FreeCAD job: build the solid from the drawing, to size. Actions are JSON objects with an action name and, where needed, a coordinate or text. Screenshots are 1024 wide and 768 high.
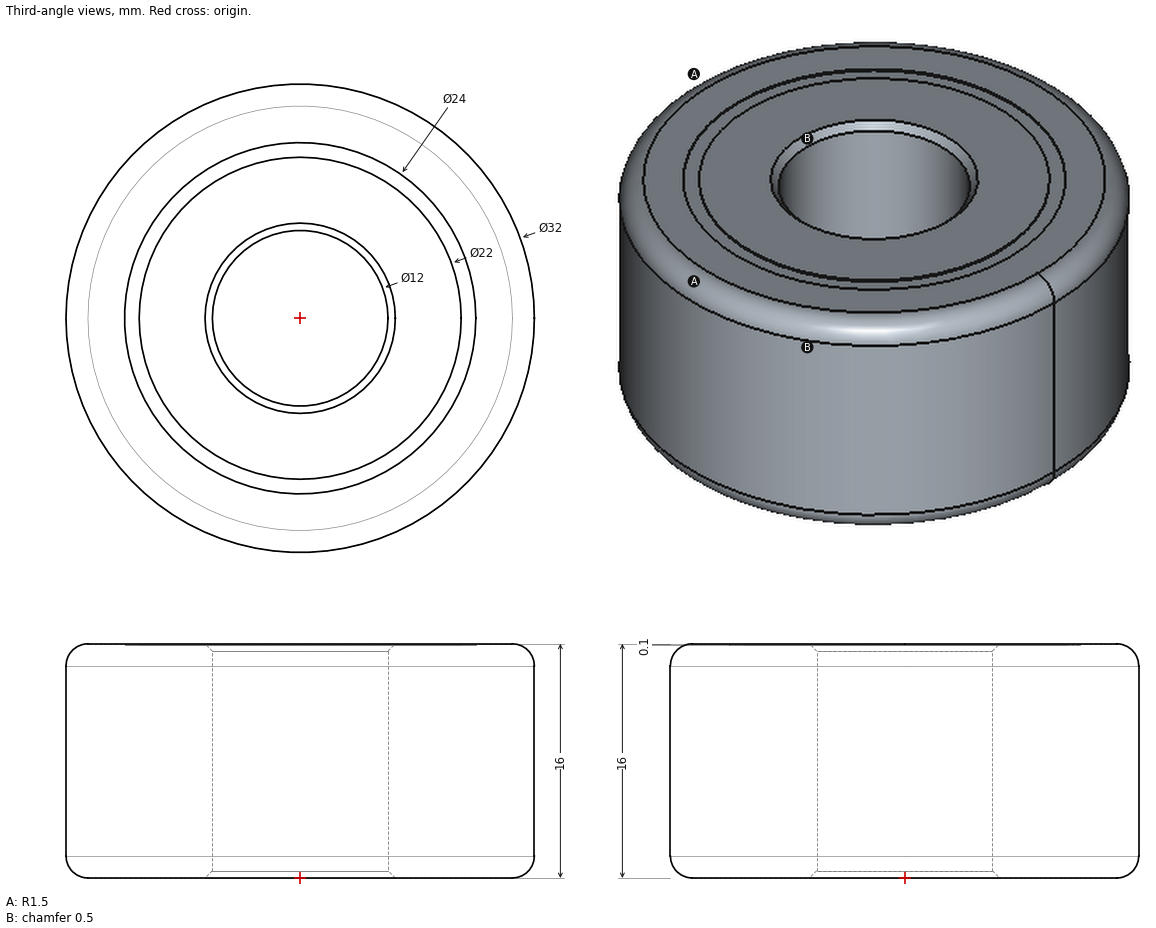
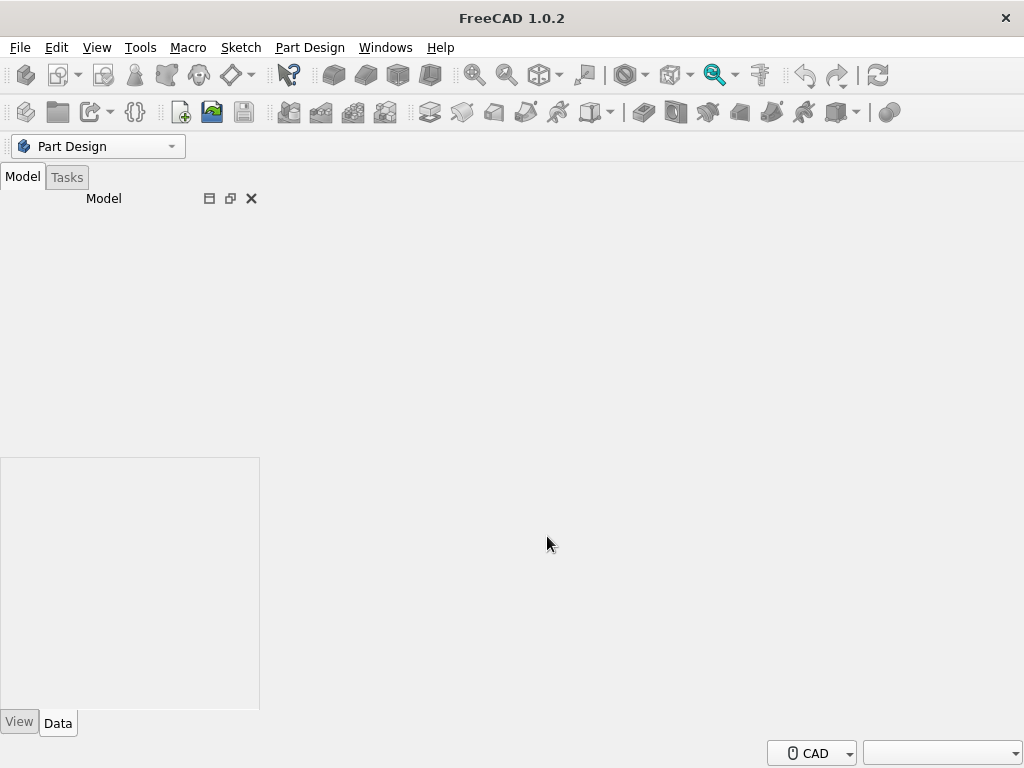
{"action": "key", "text": "ctrl+n"}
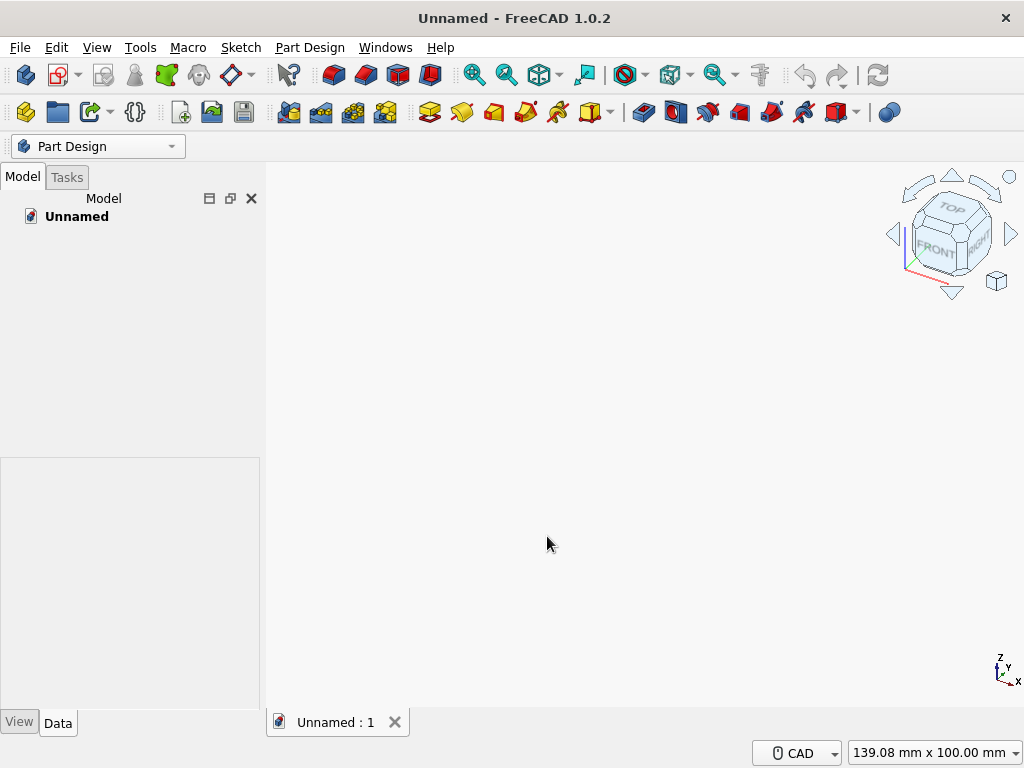
{"action": "left_click", "coordinate": [58, 76]}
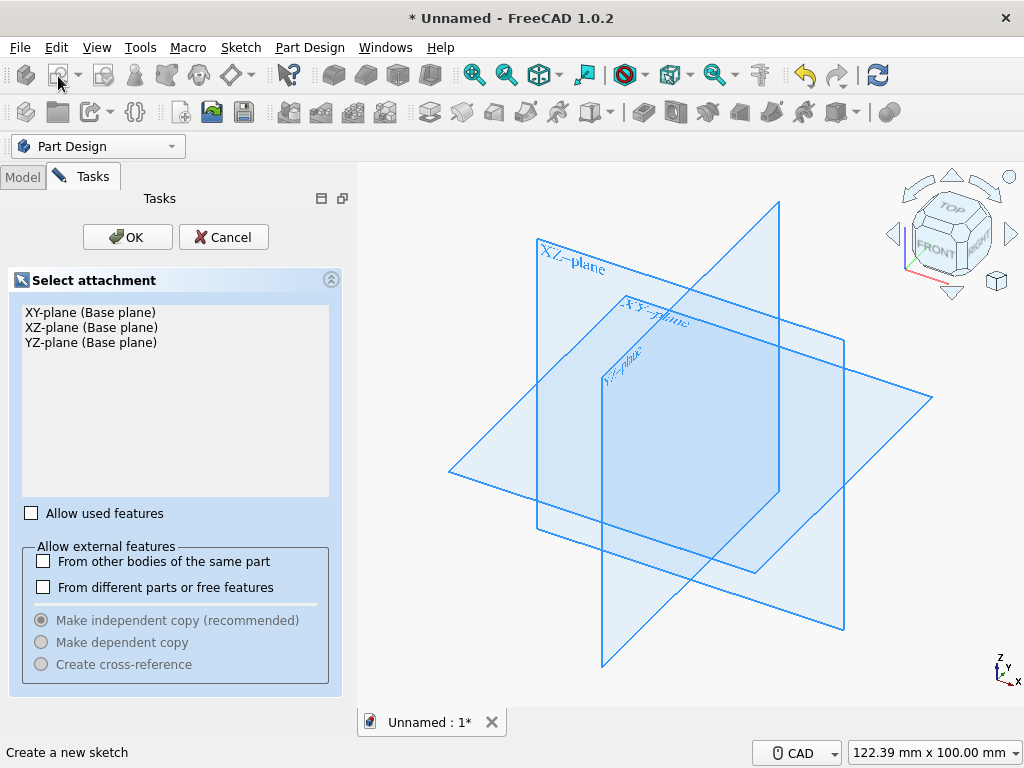
{"action": "left_click", "coordinate": [82, 312]}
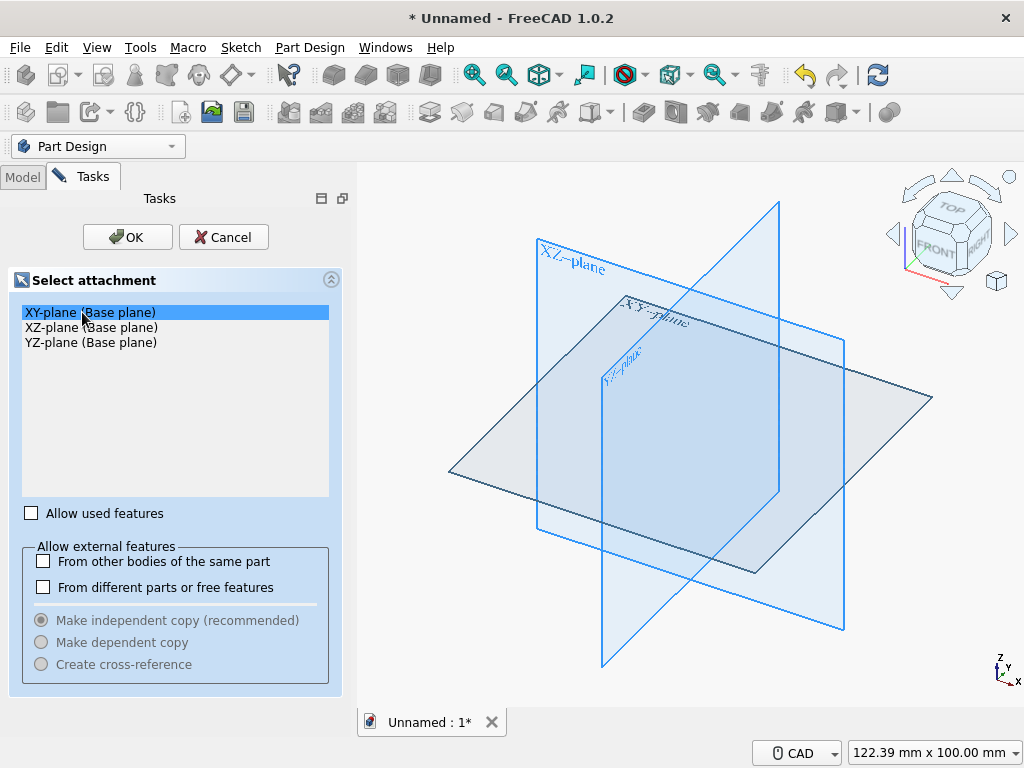
{"action": "left_click", "coordinate": [128, 237]}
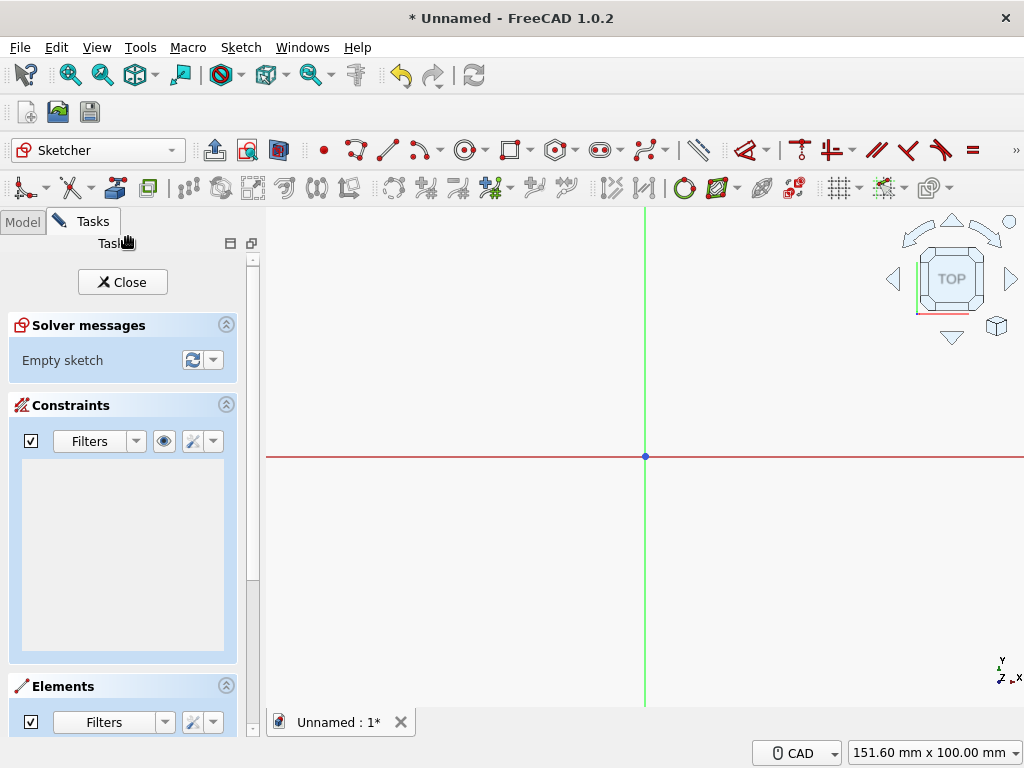
{"action": "scroll", "coordinate": [728, 457], "scroll_direction": "up", "scroll_amount": 3}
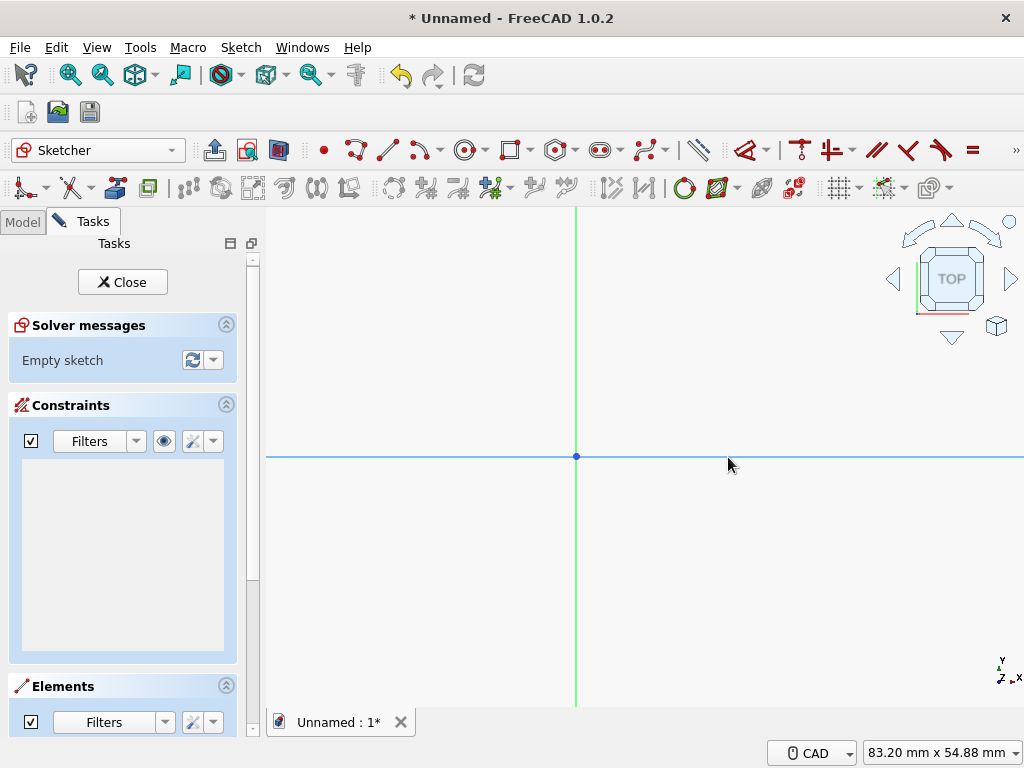
{"action": "left_click", "coordinate": [466, 150]}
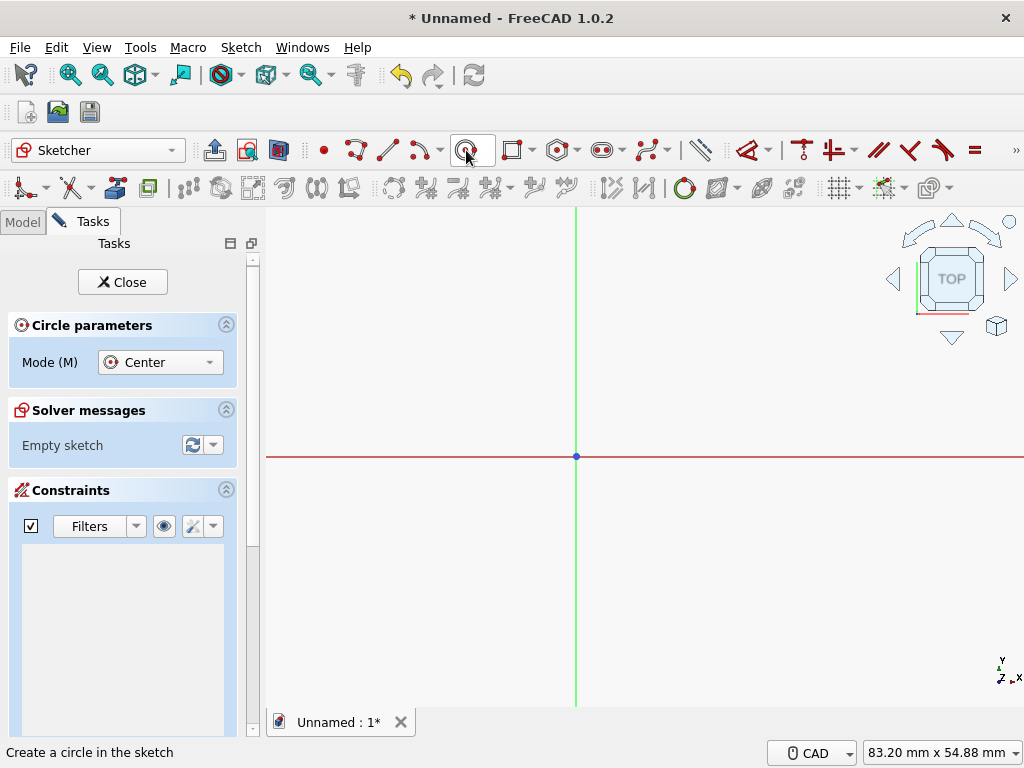
{"action": "left_click", "coordinate": [576, 457]}
{"action": "left_click", "coordinate": [679, 354]}
{"action": "key", "text": "Escape"}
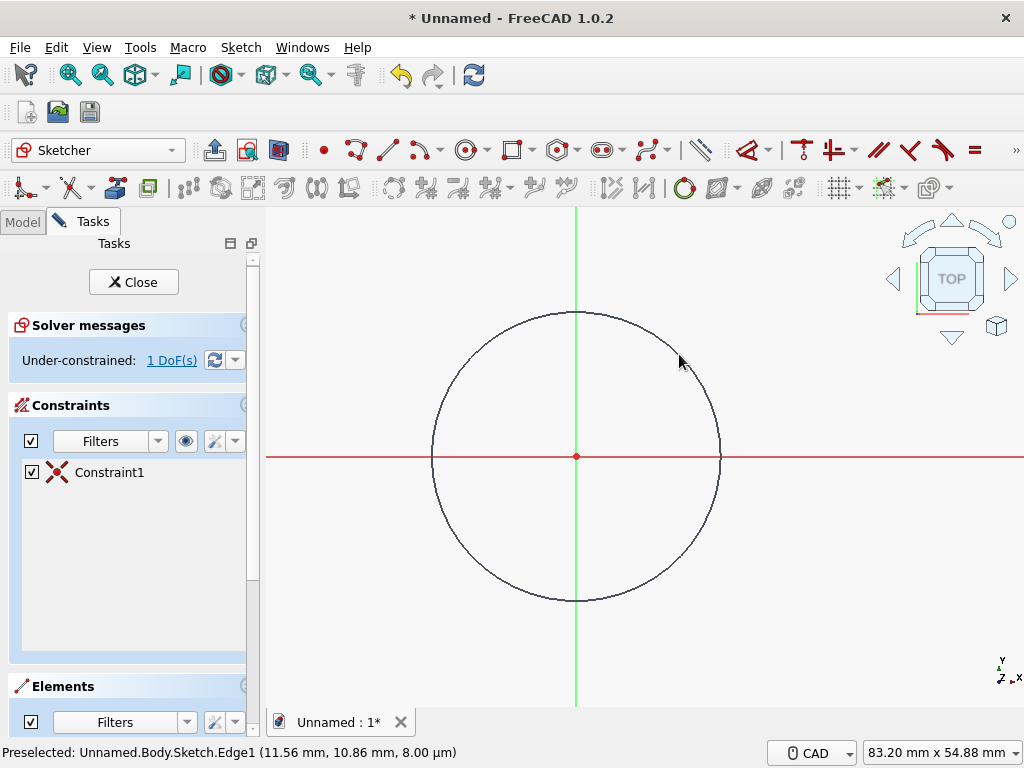
{"action": "left_click", "coordinate": [678, 354]}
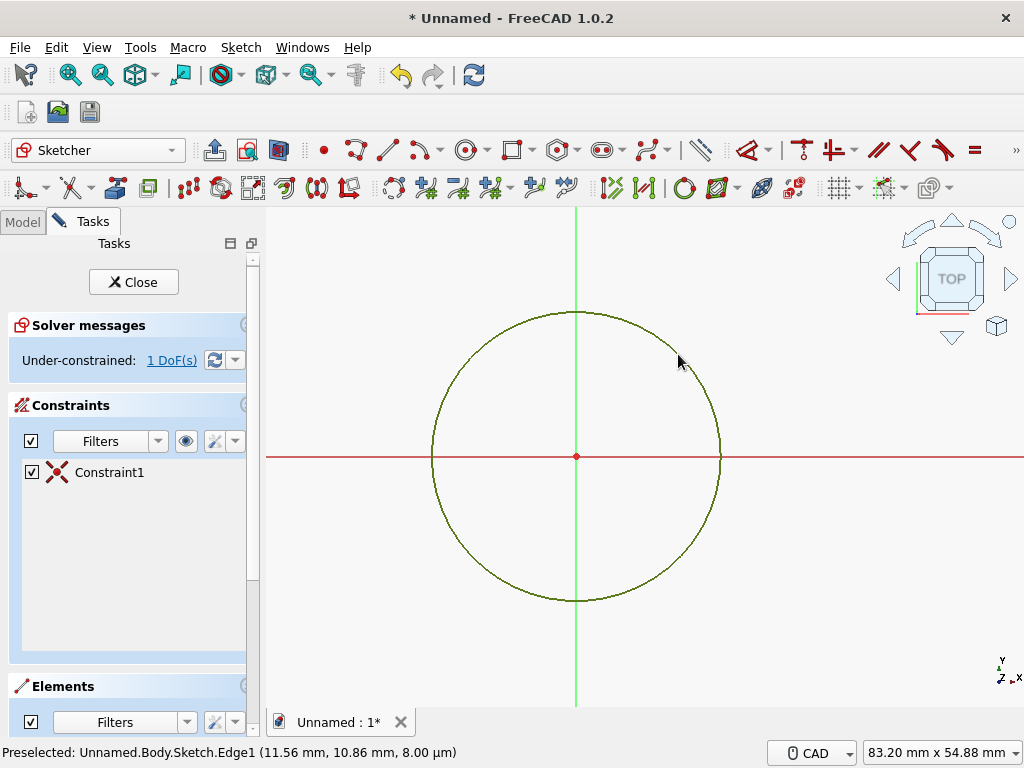
{"action": "key", "text": "k o"}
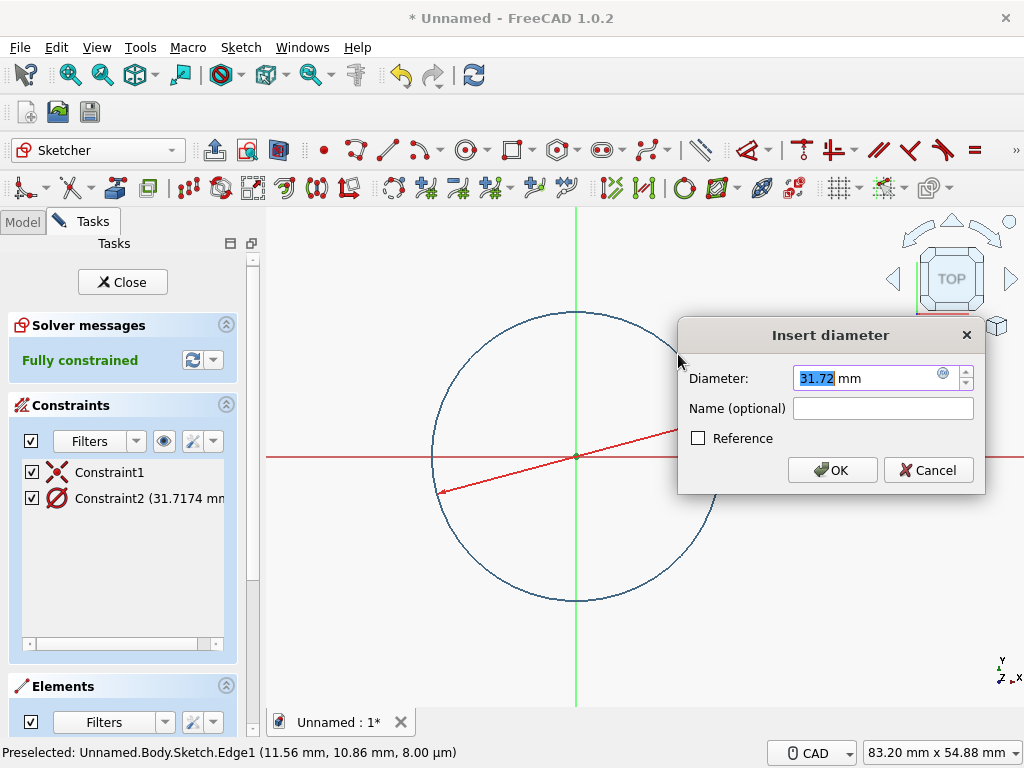
{"action": "type", "text": "32"}
{"action": "key", "text": "Return"}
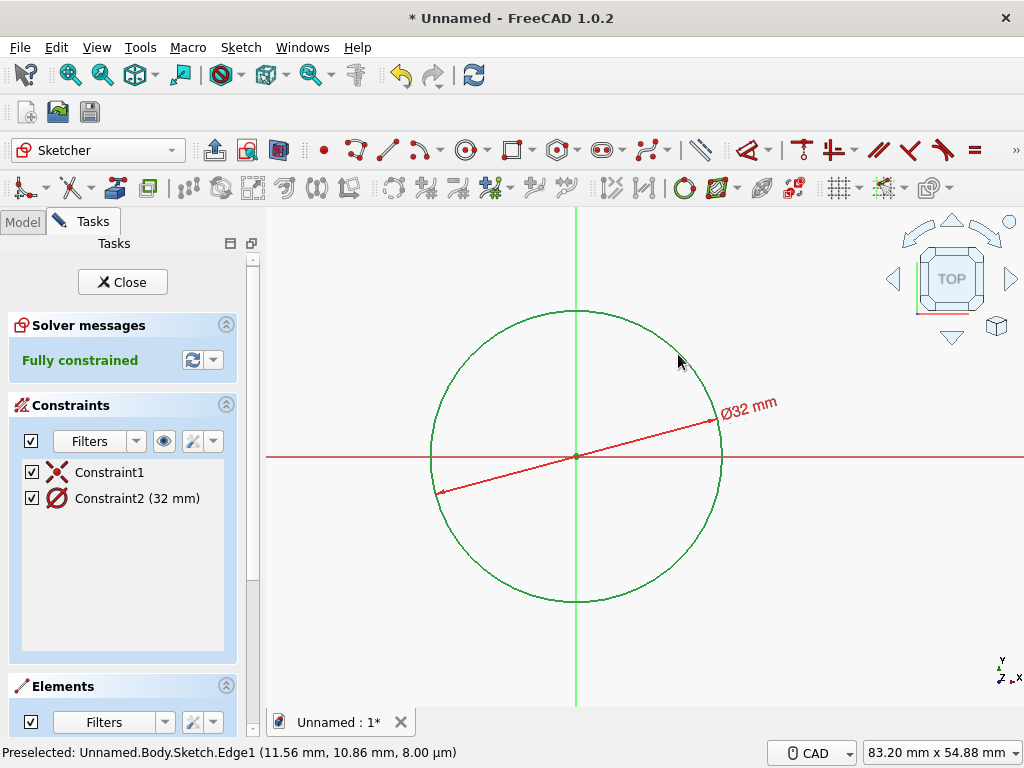
{"action": "left_click", "coordinate": [123, 282]}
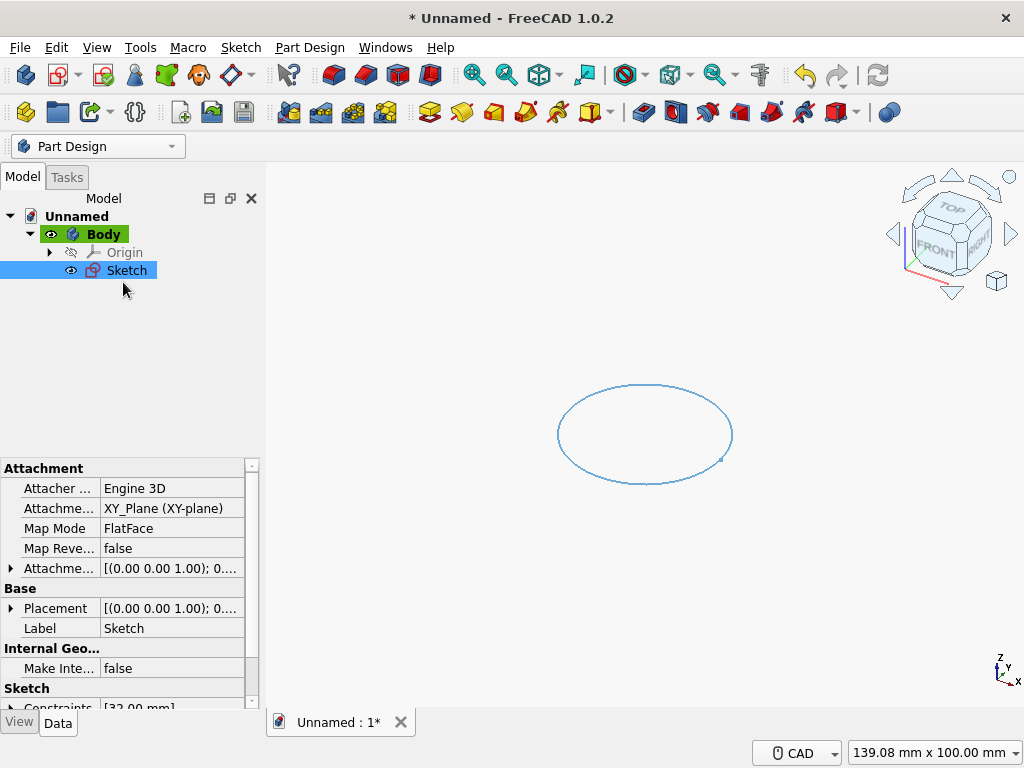
{"action": "left_click", "coordinate": [430, 112]}